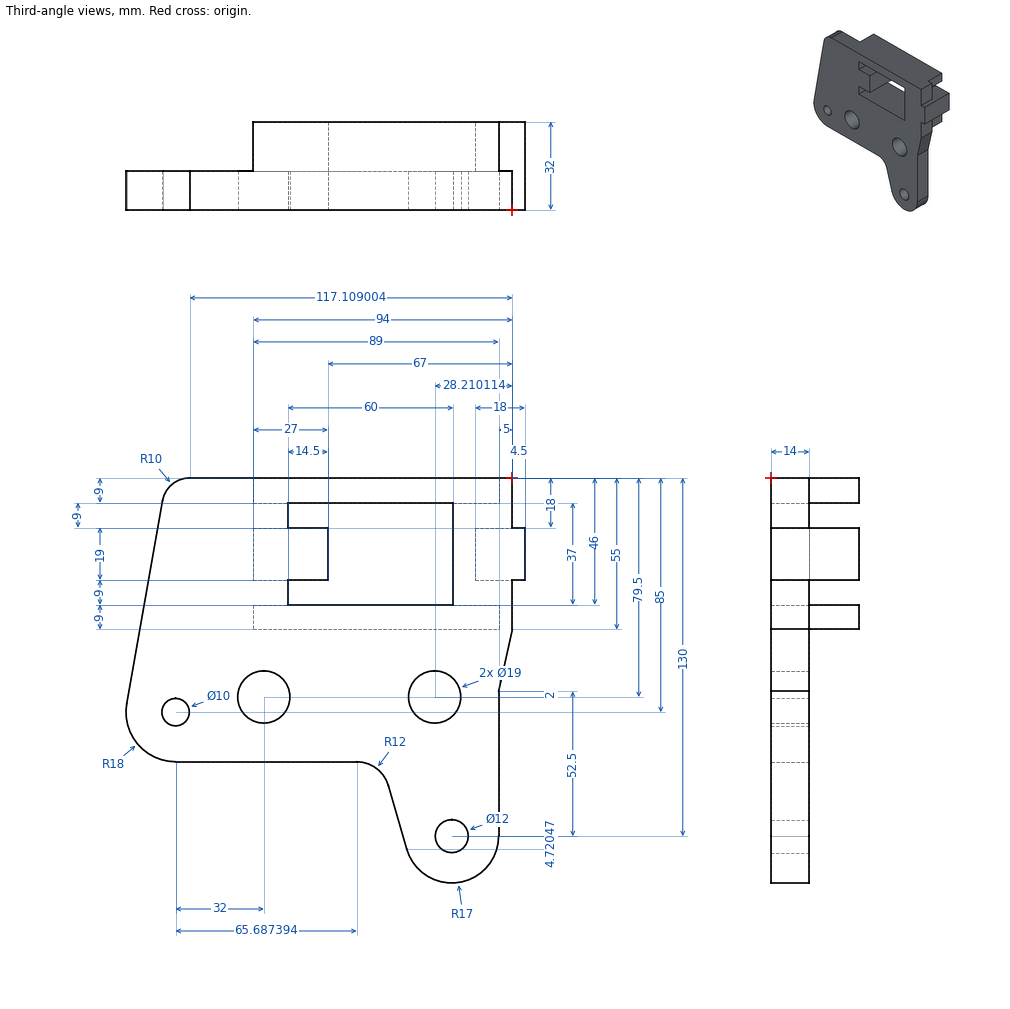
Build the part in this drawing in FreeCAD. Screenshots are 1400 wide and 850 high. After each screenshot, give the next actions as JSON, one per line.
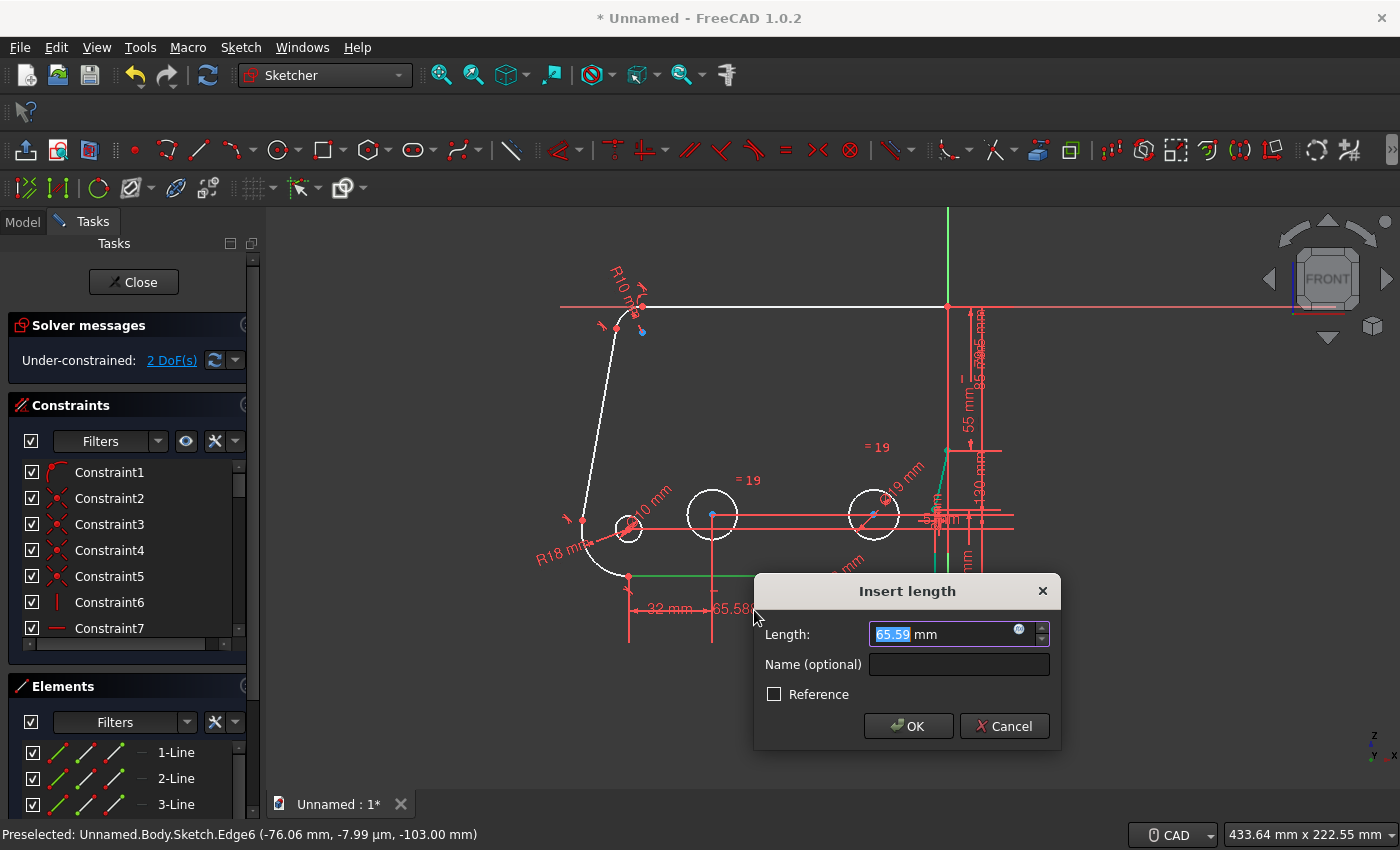
{"action": "type", "text": "65.687394"}
{"action": "key", "text": "Return"}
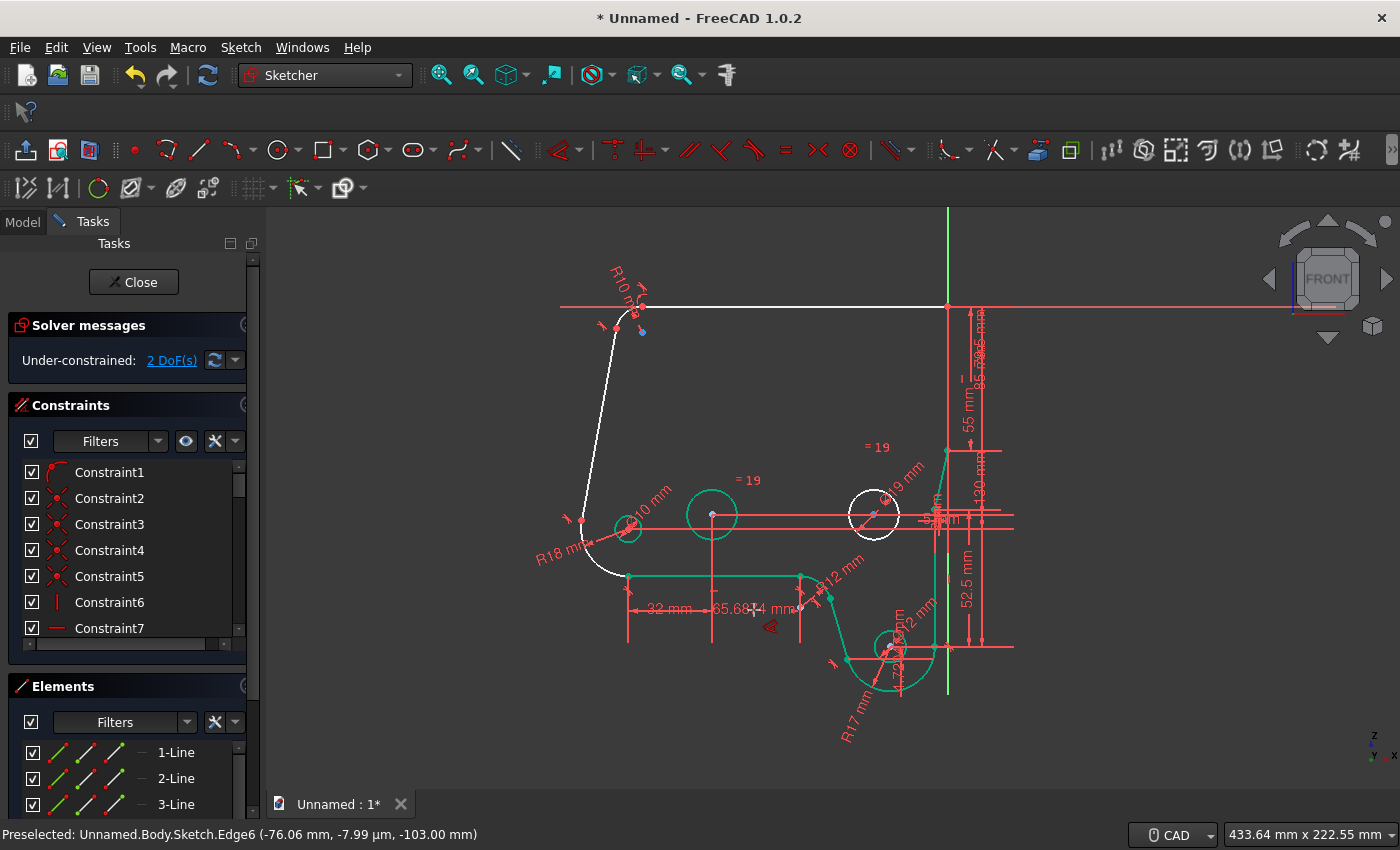
{"action": "left_click", "coordinate": [874, 515]}
{"action": "left_click", "coordinate": [911, 273]}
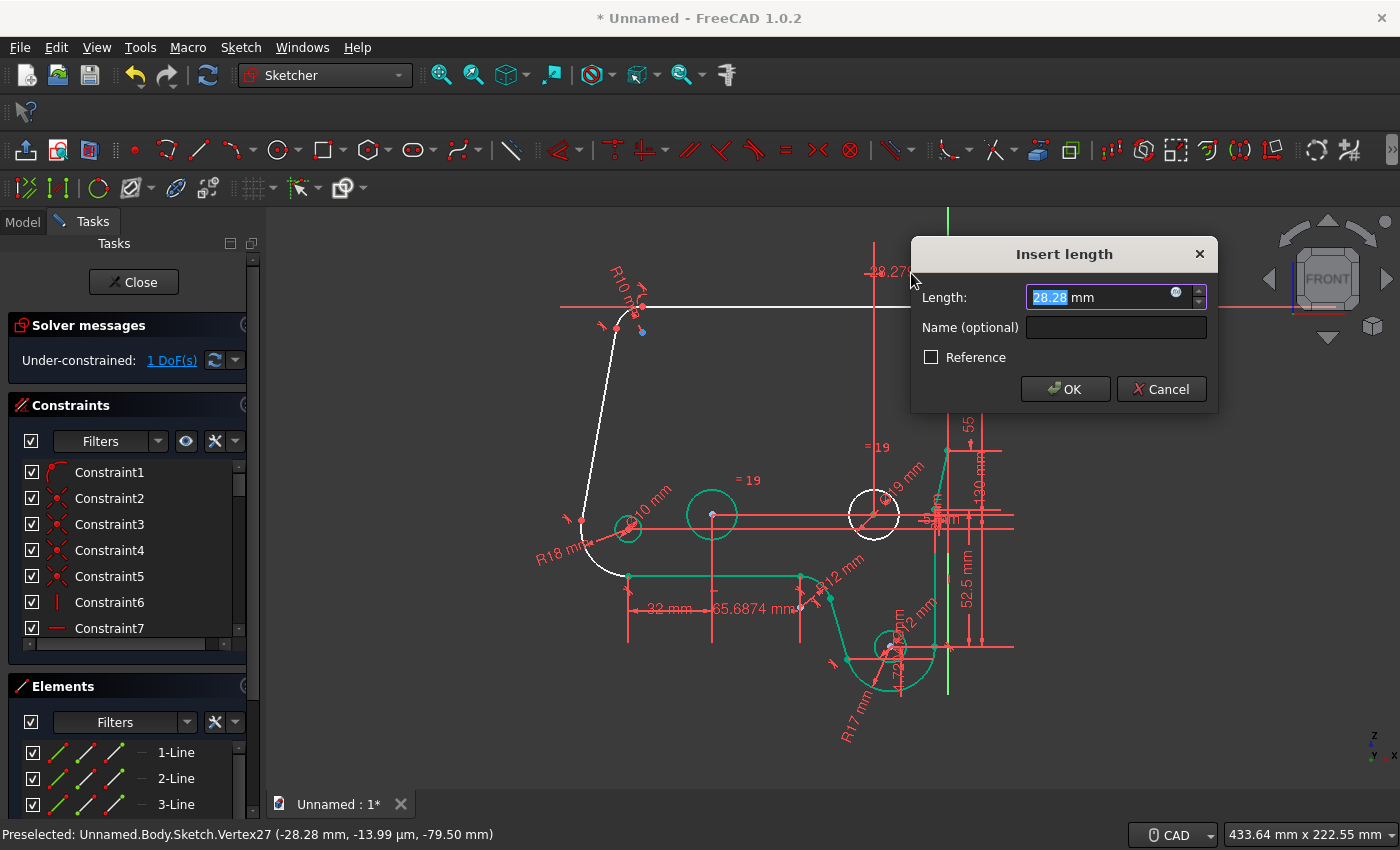
{"action": "type", "text": "28.210114"}
{"action": "key", "text": "Return"}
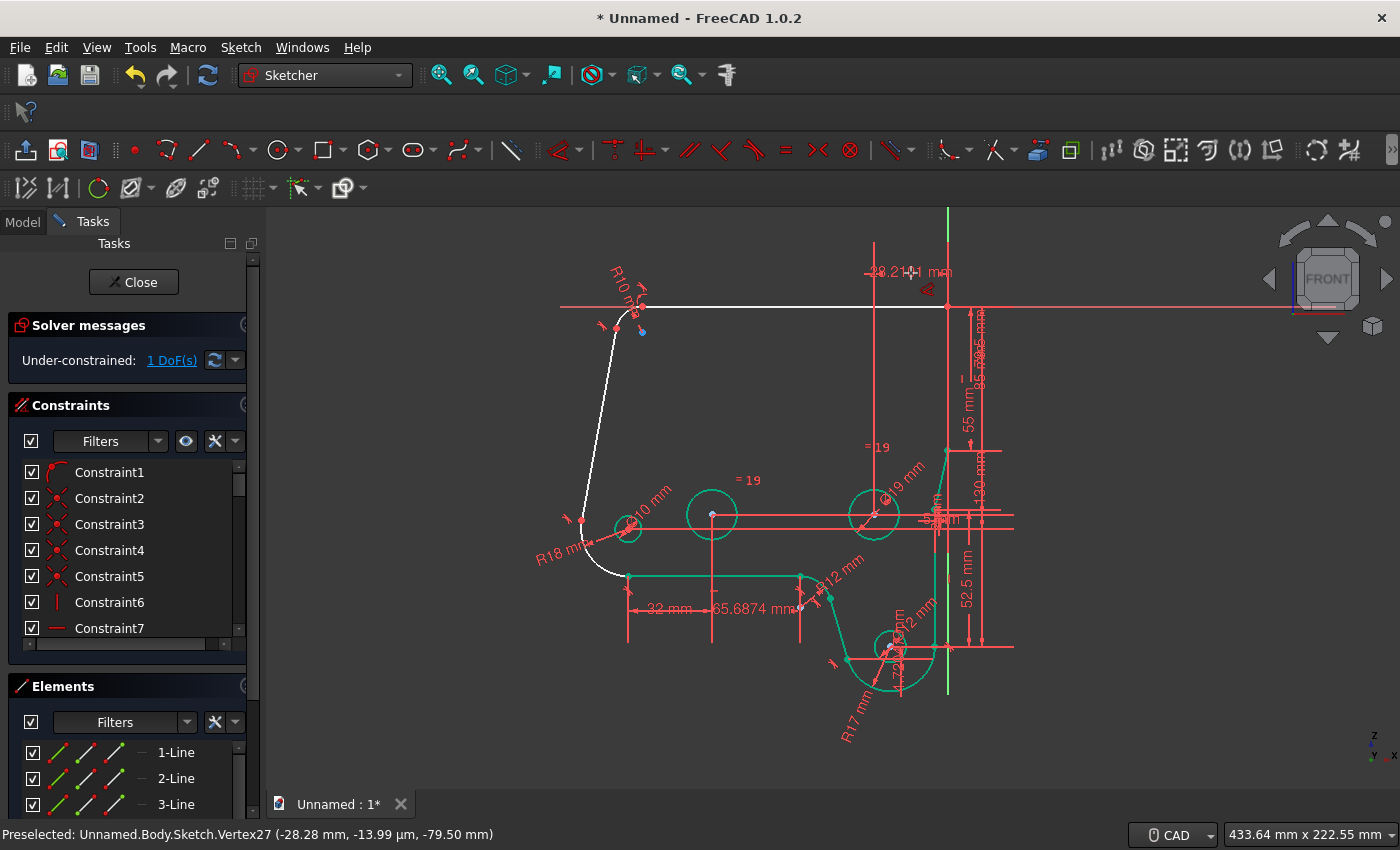
{"action": "left_click", "coordinate": [734, 307]}
{"action": "left_click", "coordinate": [795, 273]}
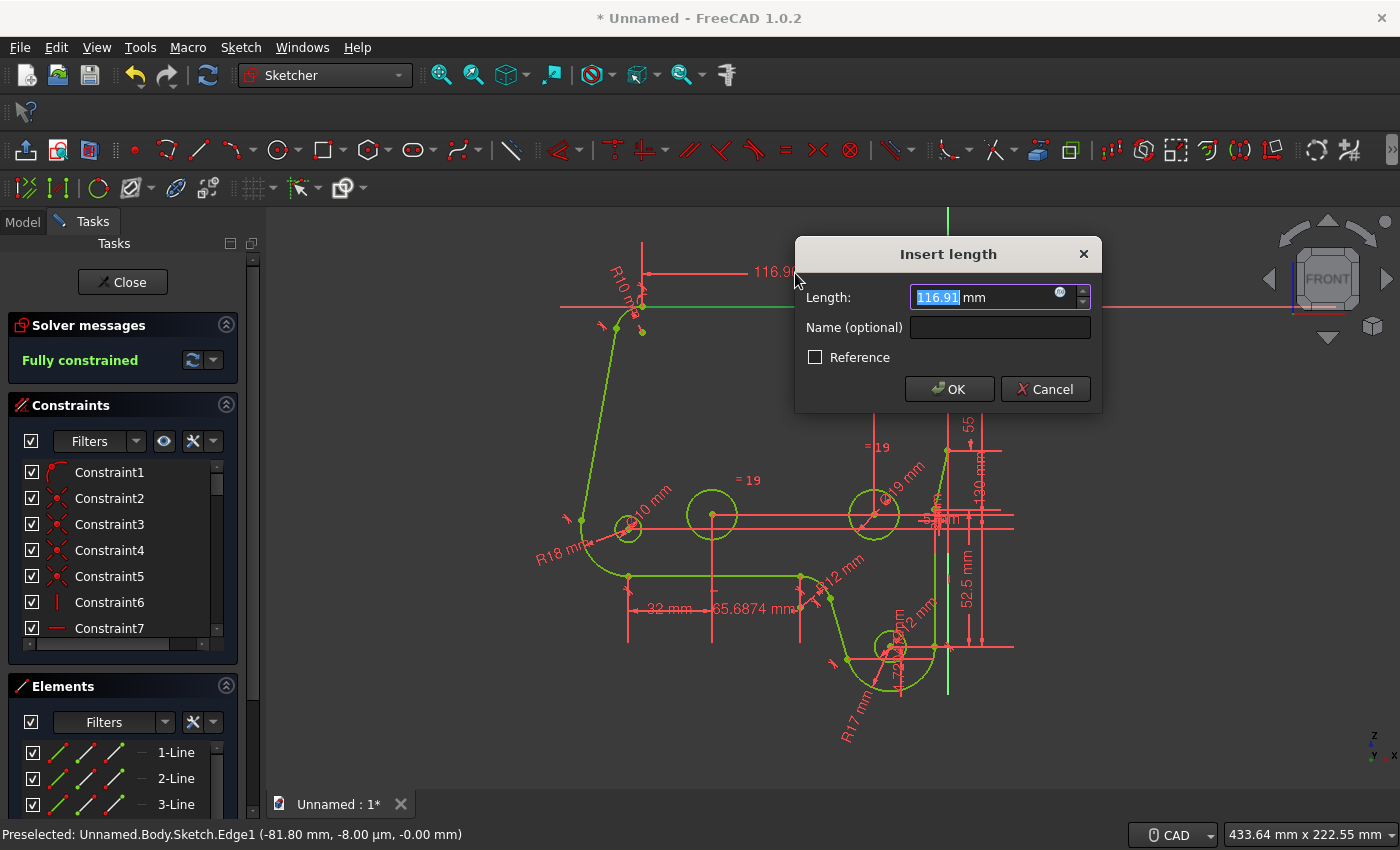
{"action": "type", "text": "117.109004"}
{"action": "key", "text": "Return"}
{"action": "key", "text": "Escape"}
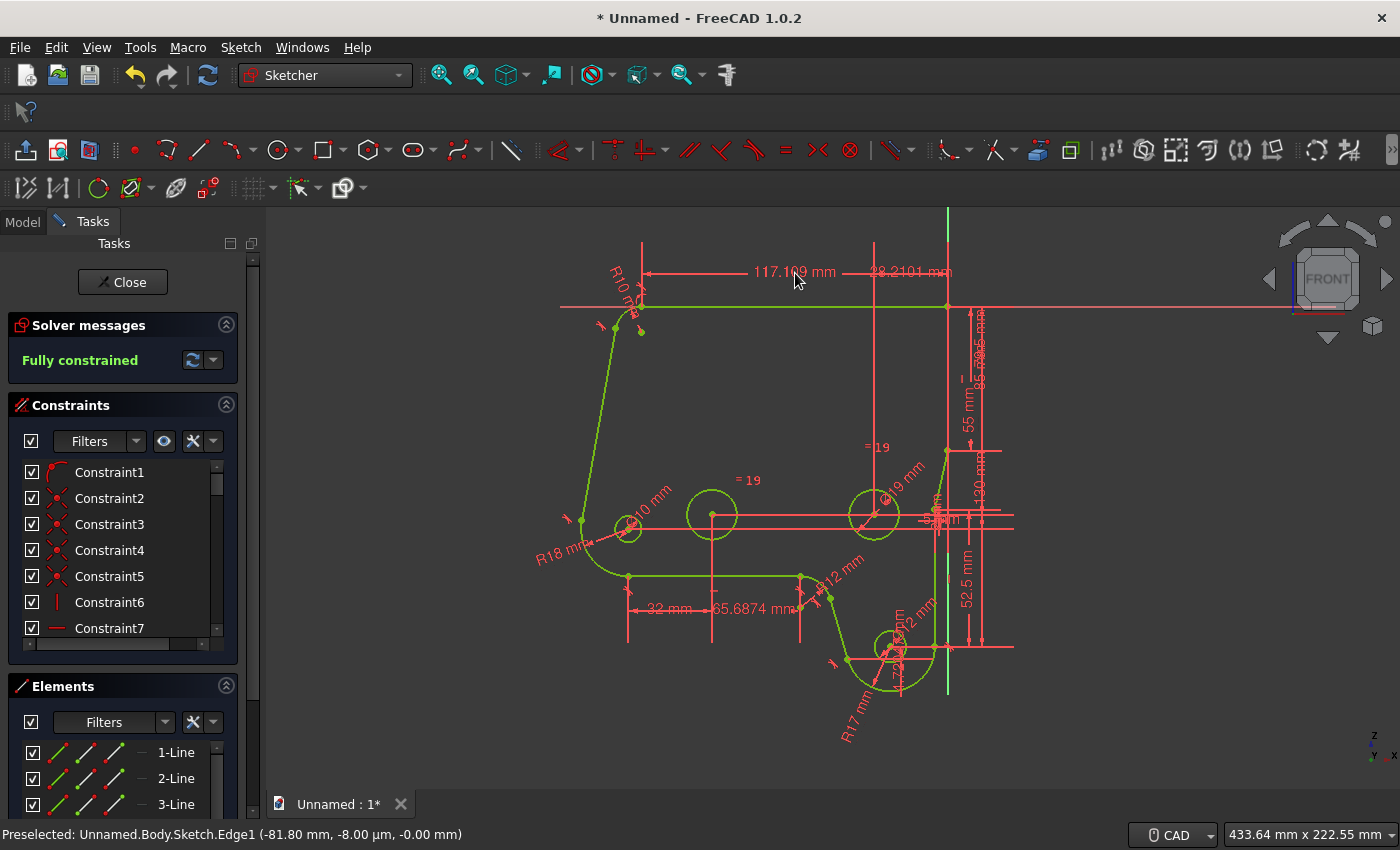
{"action": "left_click", "coordinate": [123, 282]}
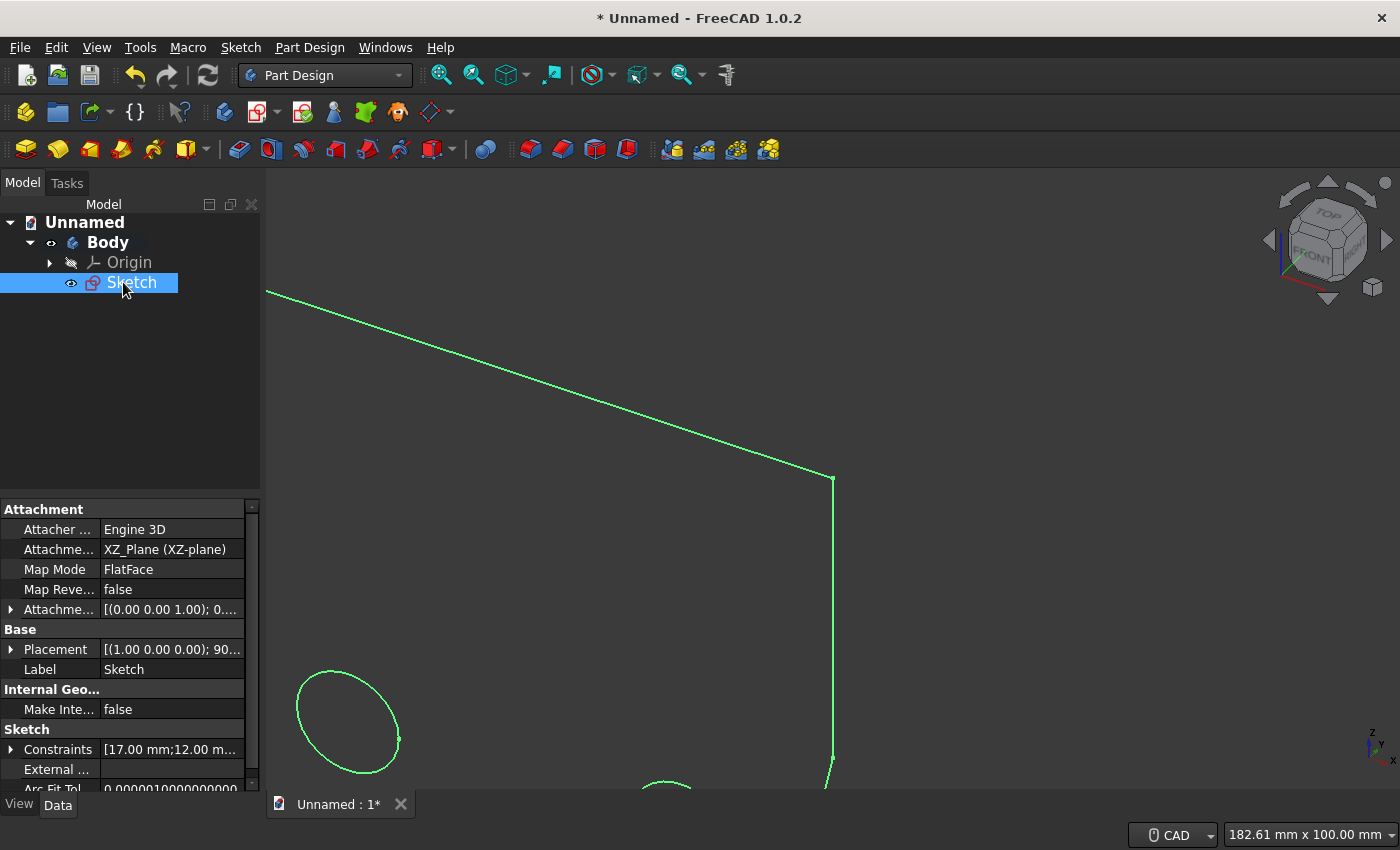
{"action": "left_click", "coordinate": [26, 150]}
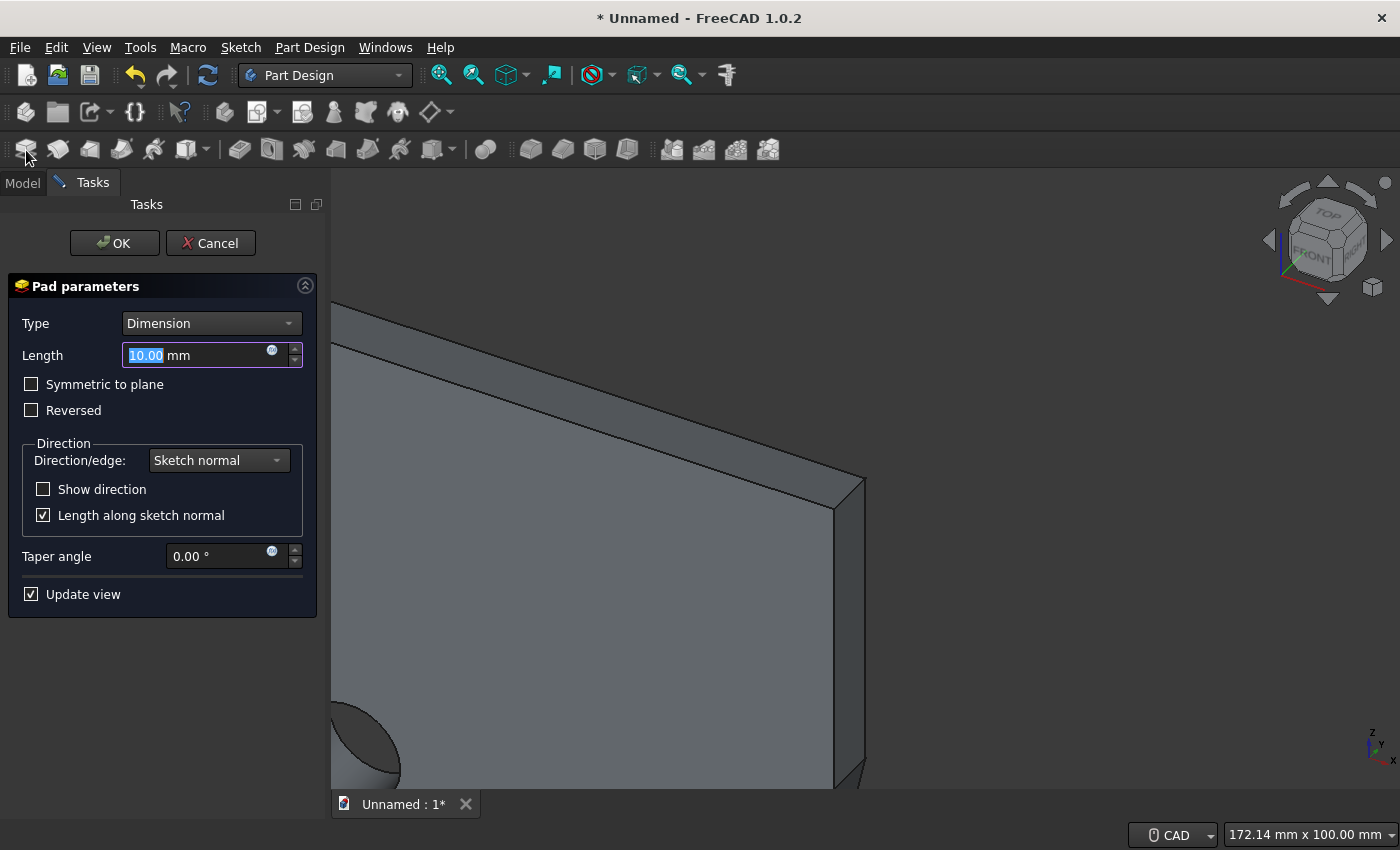
{"action": "type", "text": "14"}
{"action": "key", "text": "Tab"}